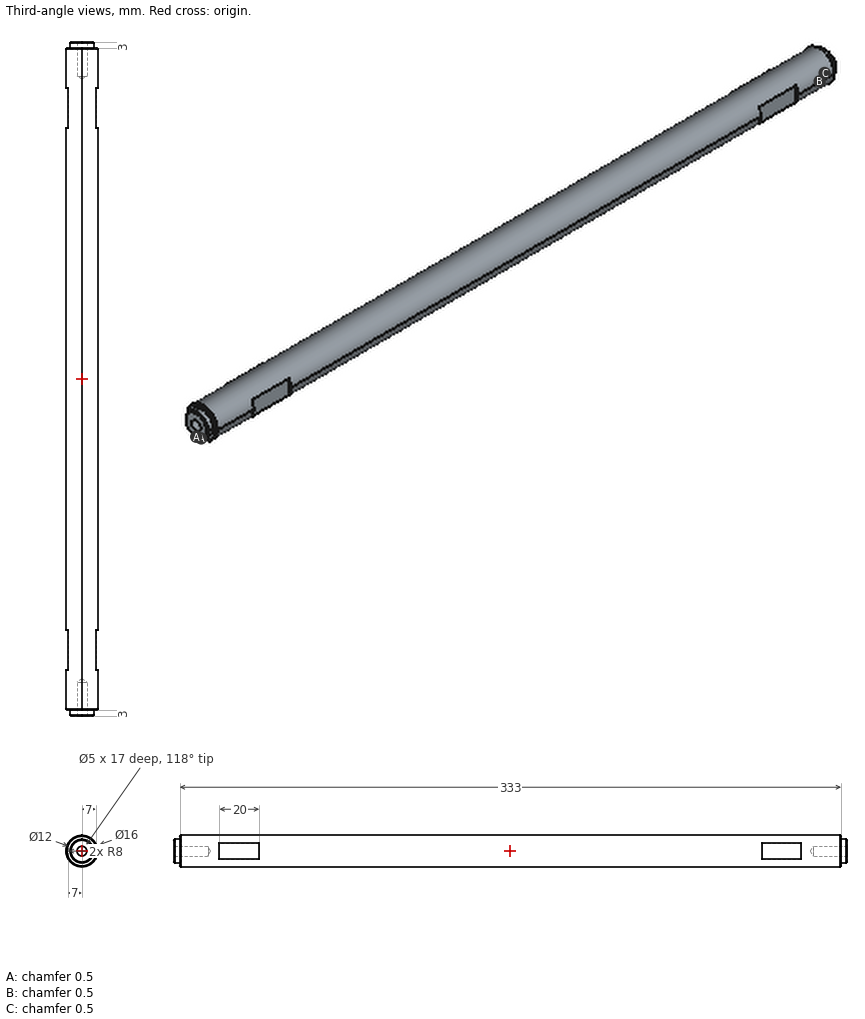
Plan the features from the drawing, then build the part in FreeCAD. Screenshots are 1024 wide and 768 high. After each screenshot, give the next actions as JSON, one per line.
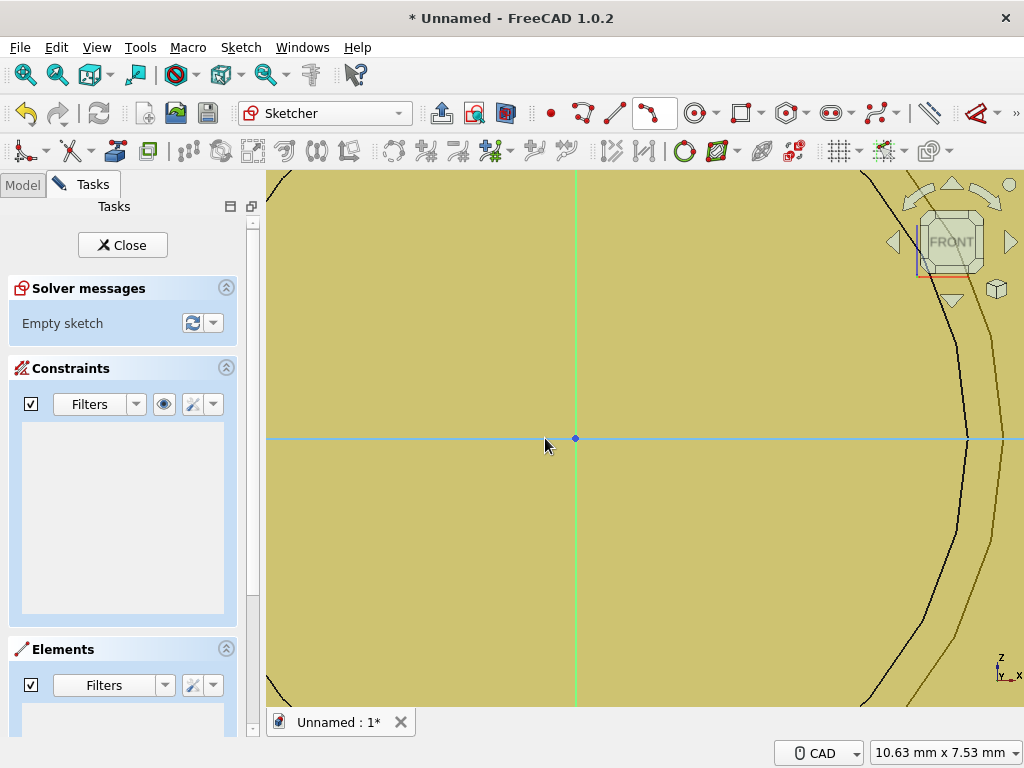
{"action": "key", "text": "g c"}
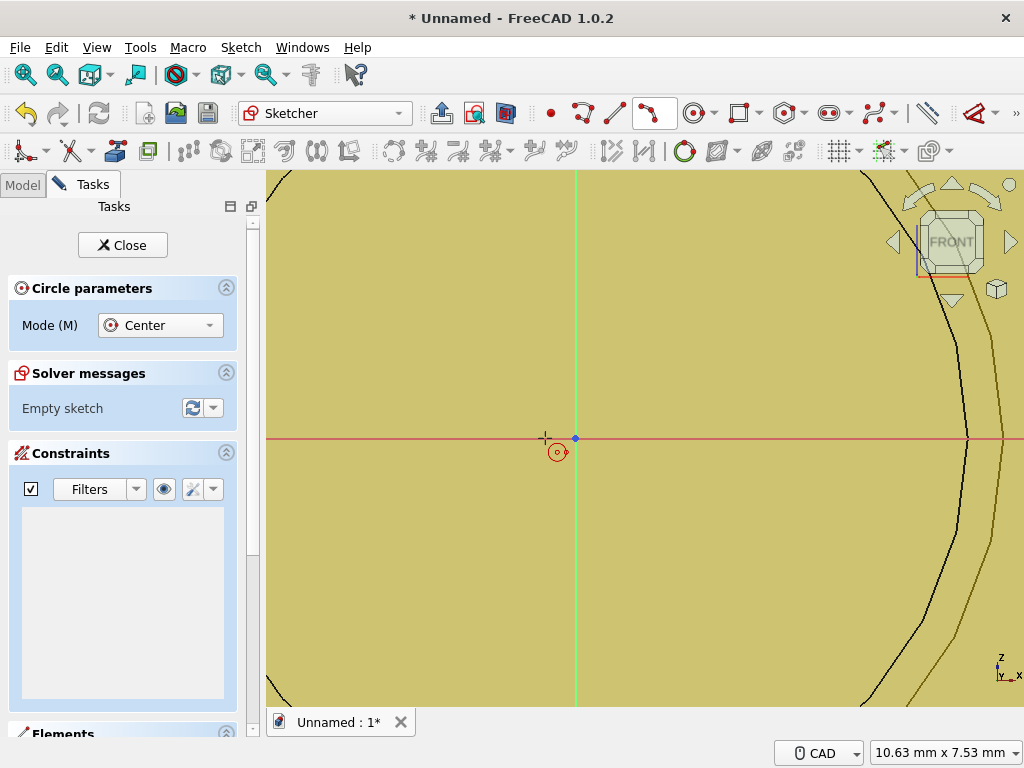
{"action": "left_click", "coordinate": [576, 438]}
{"action": "left_click", "coordinate": [702, 312]}
{"action": "key", "text": "Escape"}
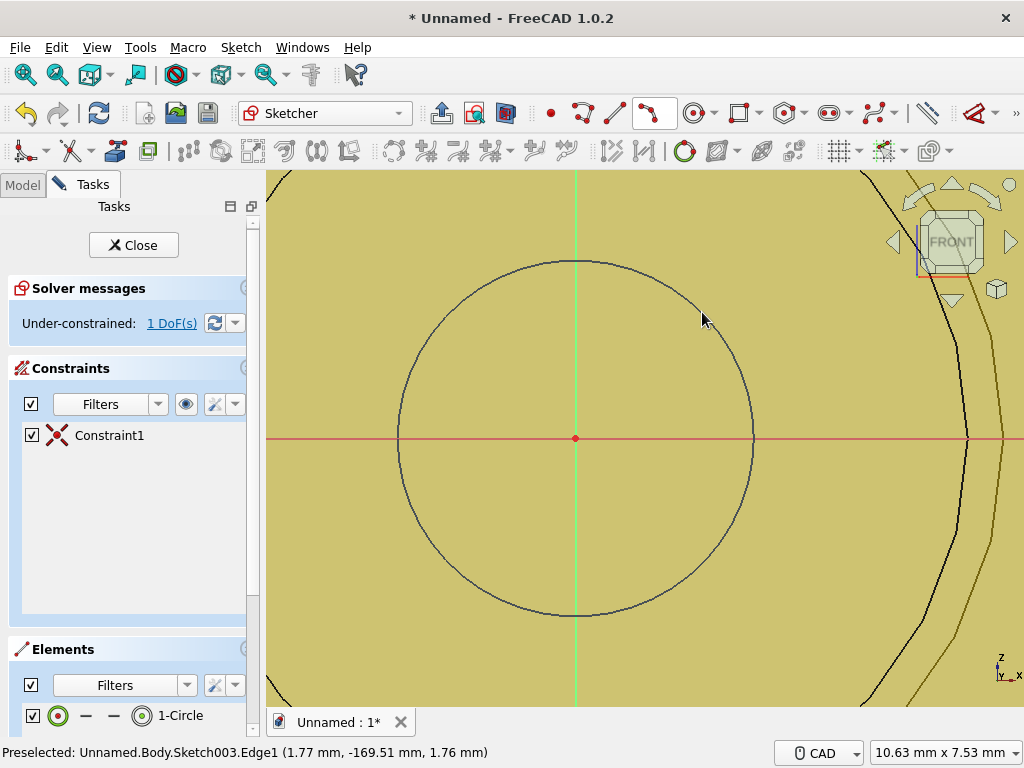
{"action": "key", "text": "d"}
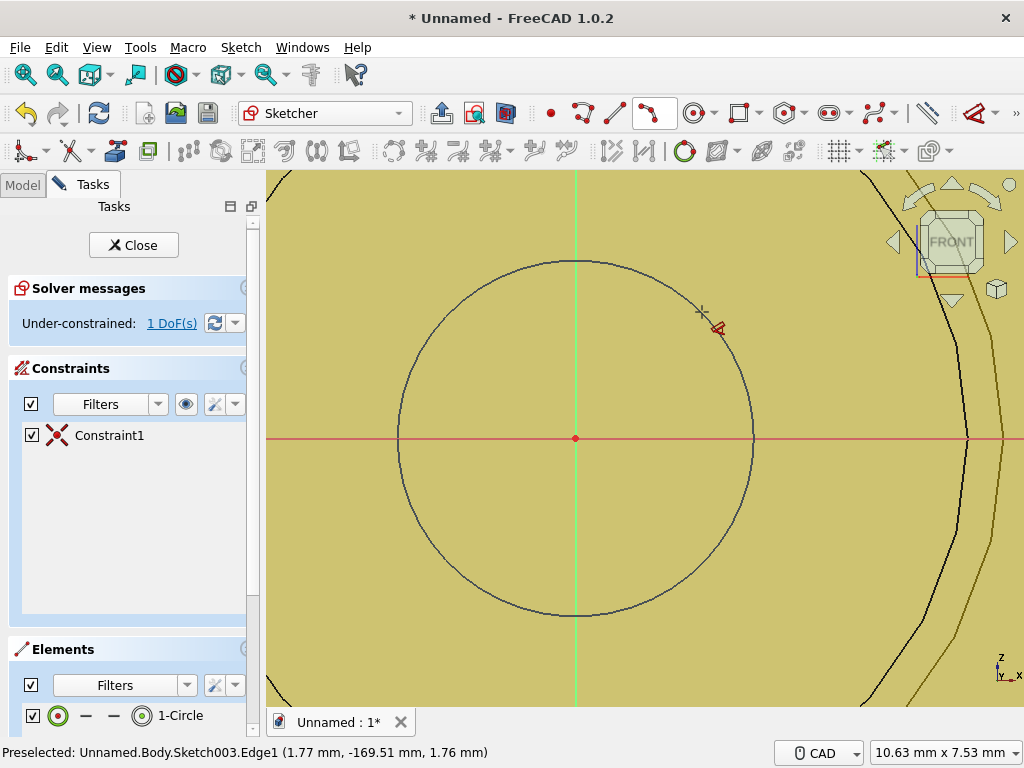
{"action": "left_click", "coordinate": [701, 312]}
{"action": "left_click", "coordinate": [724, 289]}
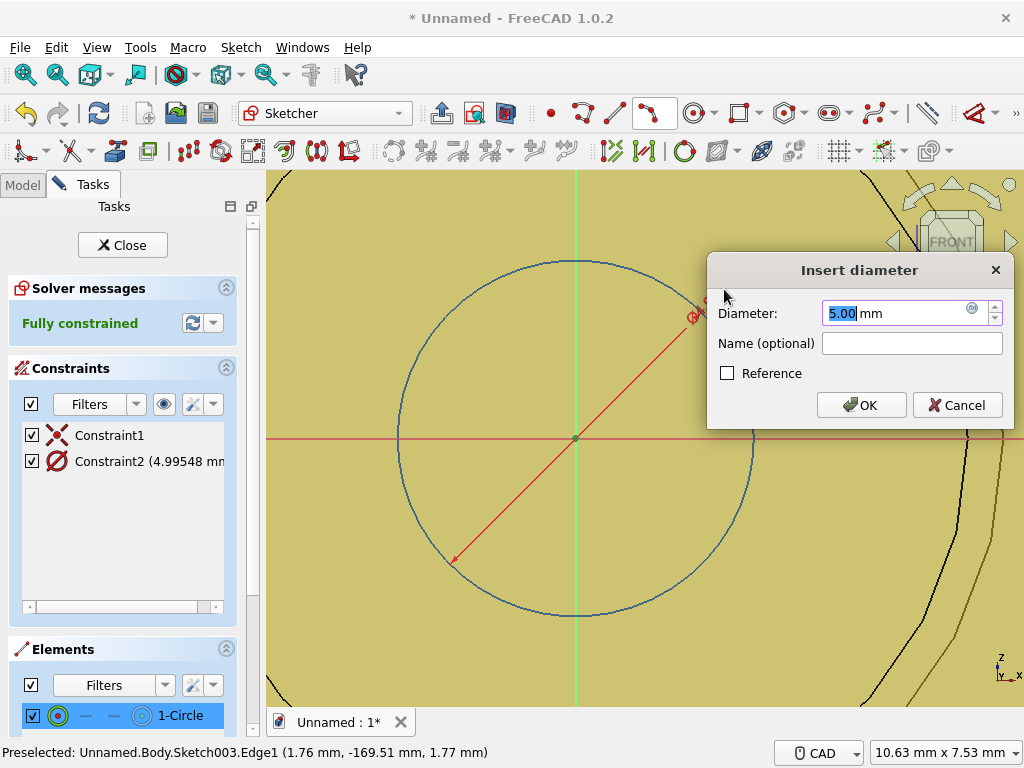
{"action": "type", "text": "5"}
{"action": "key", "text": "Return"}
{"action": "key", "text": "Escape"}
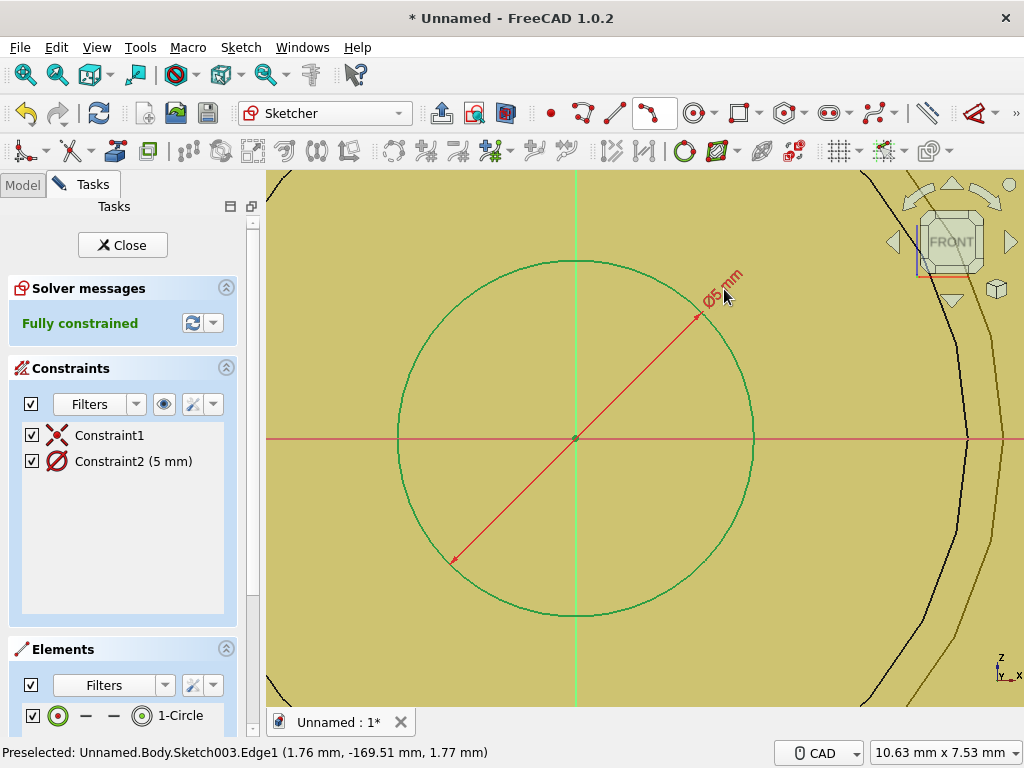
{"action": "left_click", "coordinate": [123, 245]}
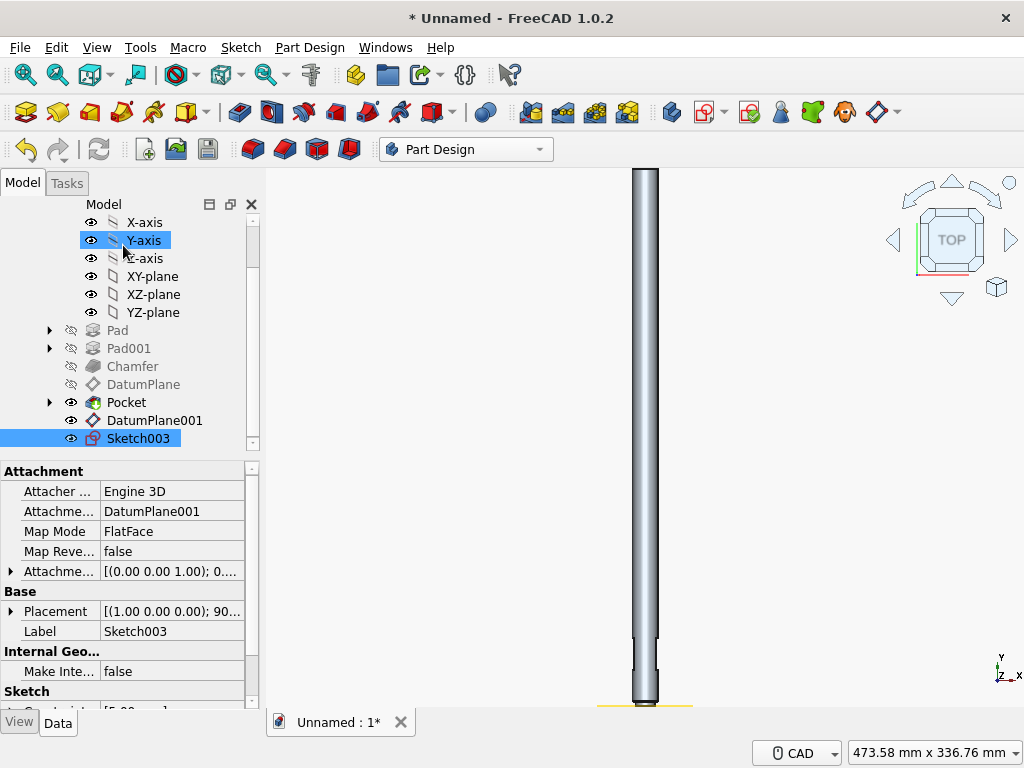
{"action": "left_click", "coordinate": [272, 112]}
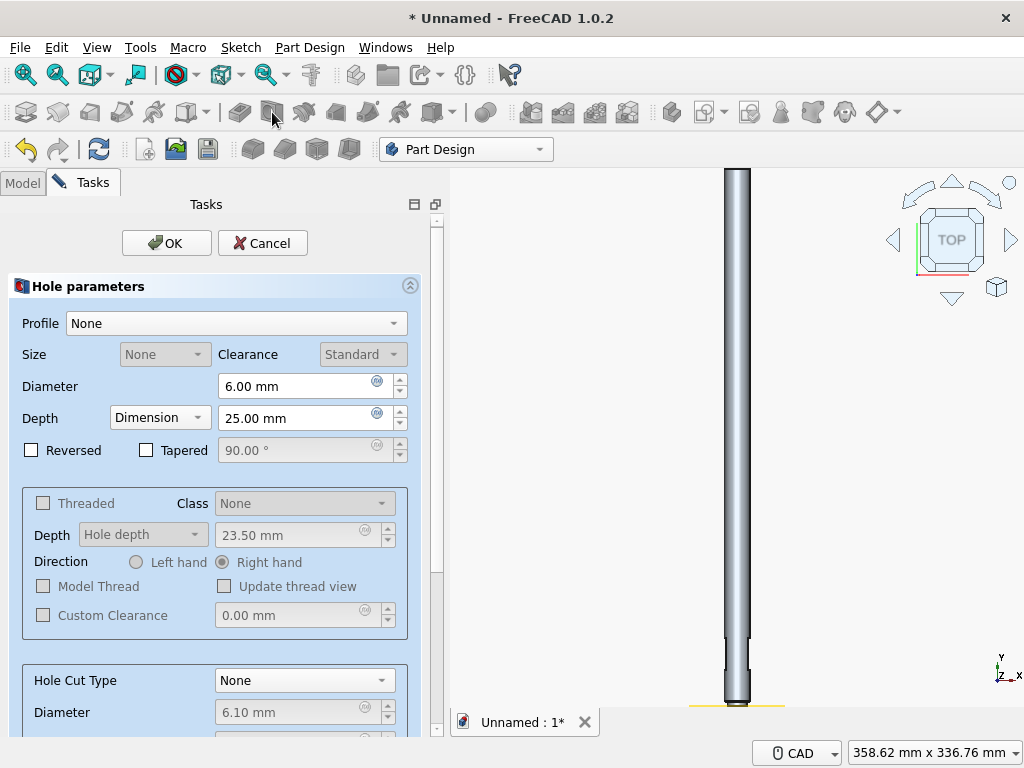
{"action": "triple_click", "coordinate": [305, 386]}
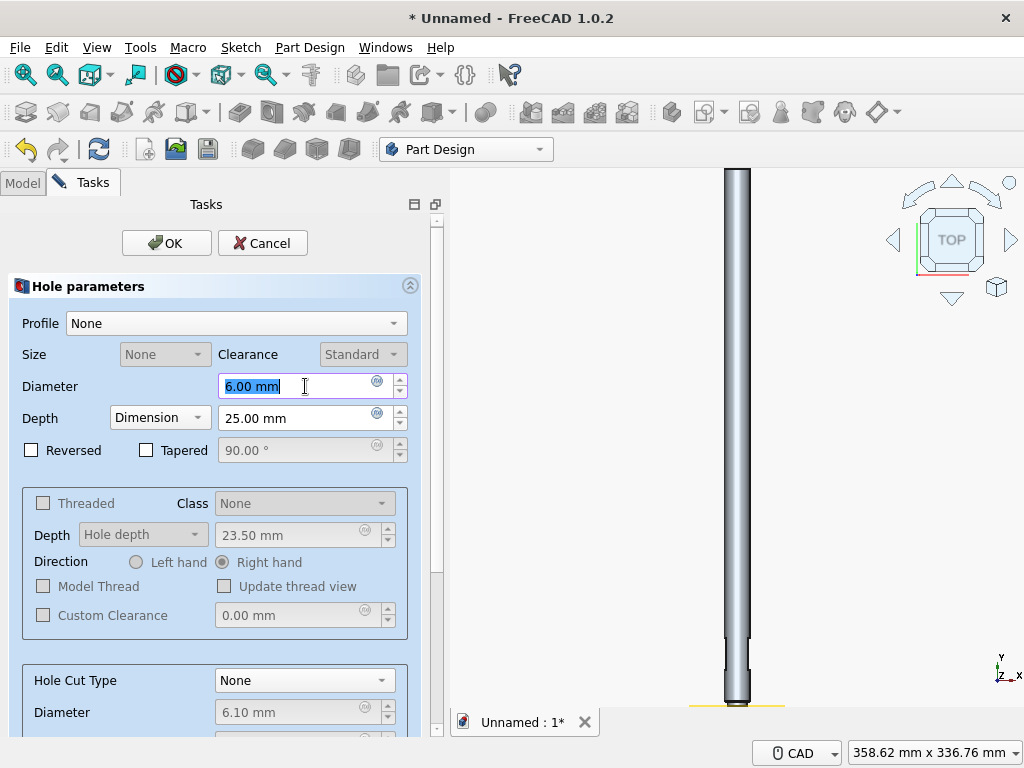
{"action": "type", "text": "5"}
{"action": "key", "text": "Tab"}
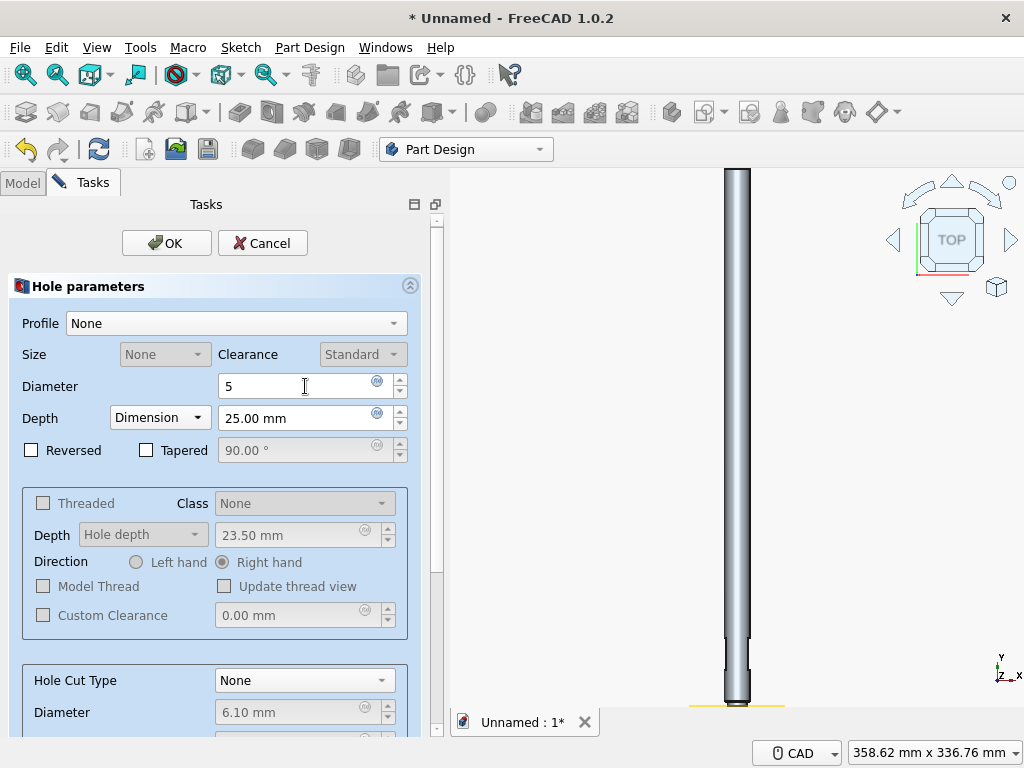
{"action": "triple_click", "coordinate": [305, 418]}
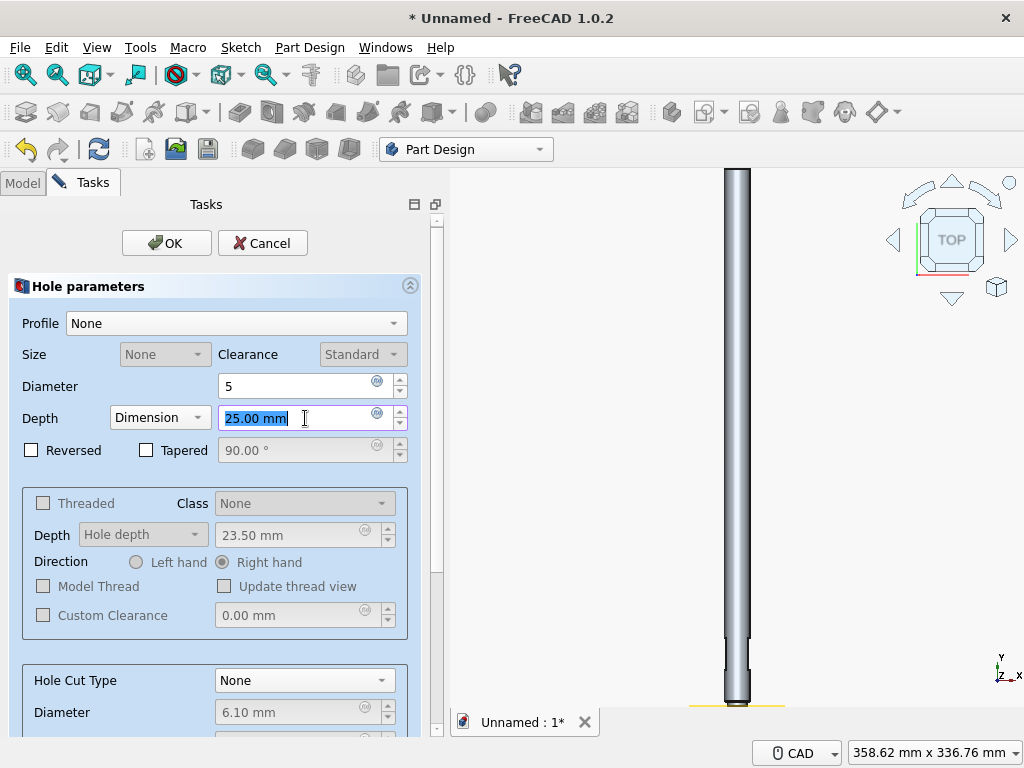
{"action": "type", "text": "17"}
{"action": "key", "text": "Tab"}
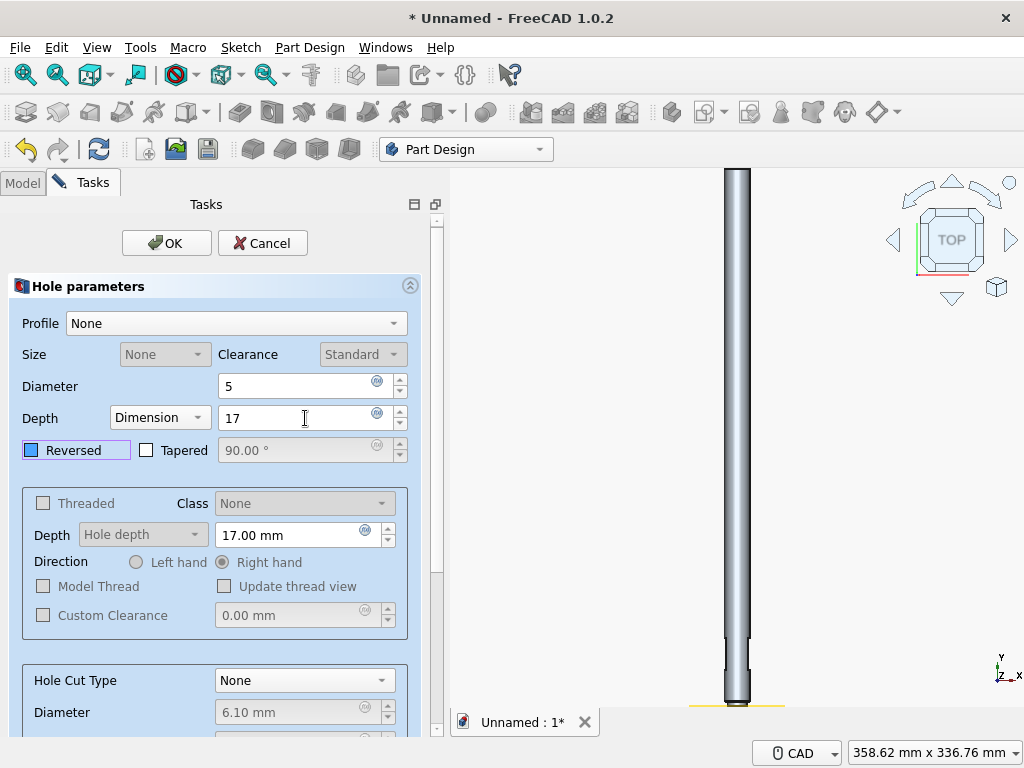
{"action": "left_click", "coordinate": [167, 243]}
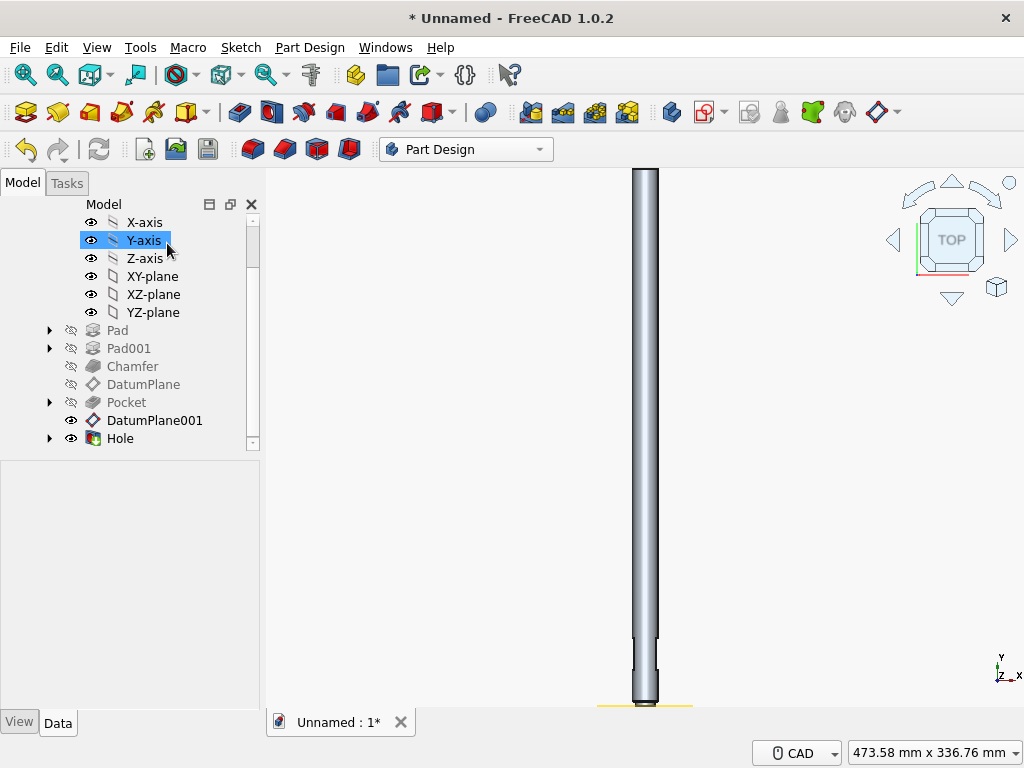
{"action": "left_click", "coordinate": [116, 420]}
{"action": "key", "text": "space"}